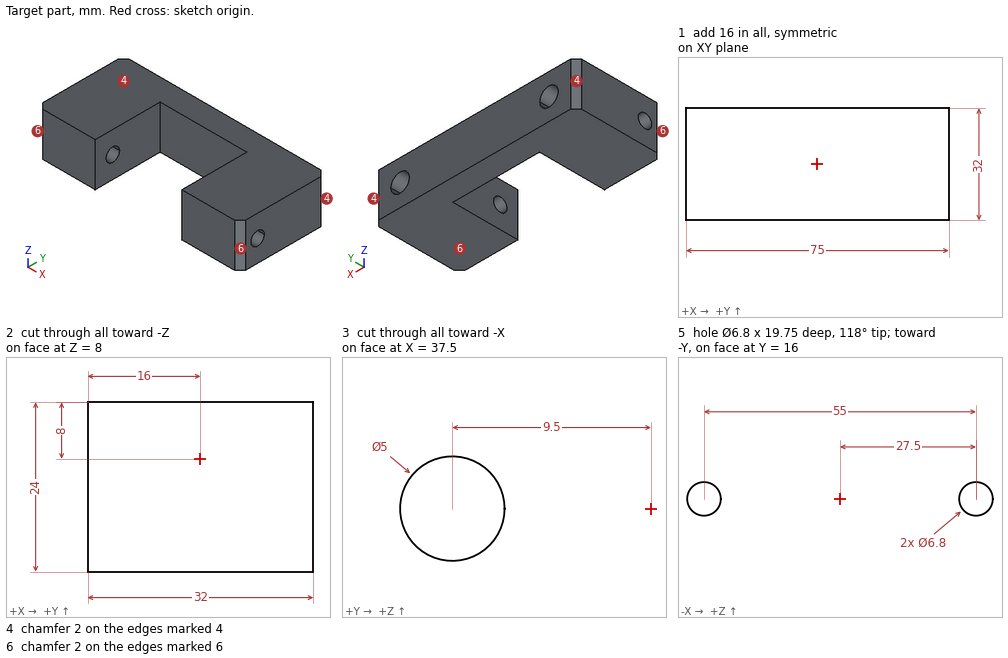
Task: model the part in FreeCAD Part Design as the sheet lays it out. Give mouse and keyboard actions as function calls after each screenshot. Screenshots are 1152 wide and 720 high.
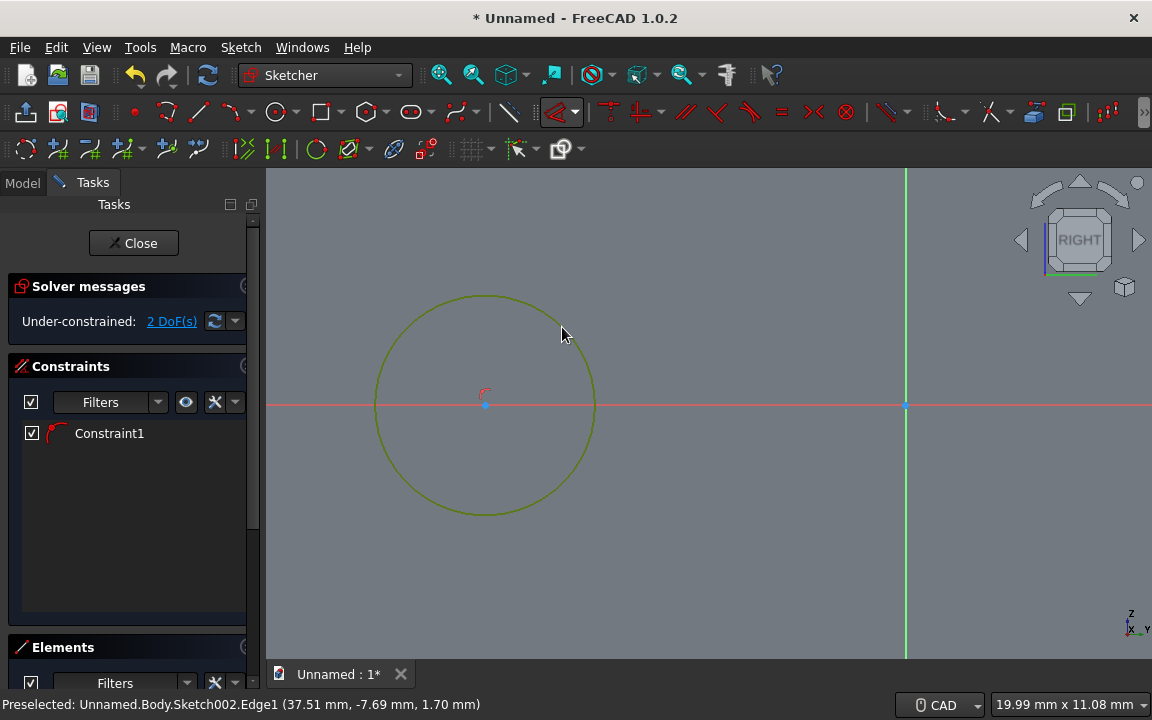
key(k)
key(o)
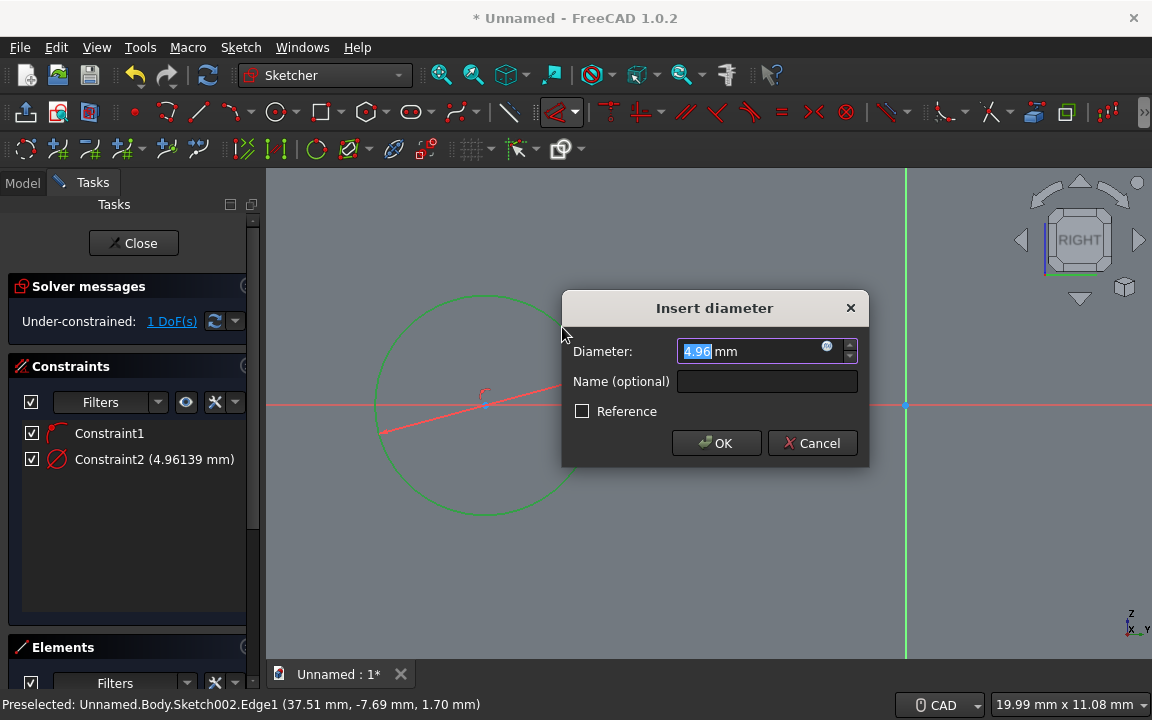
text(5)
key(Return)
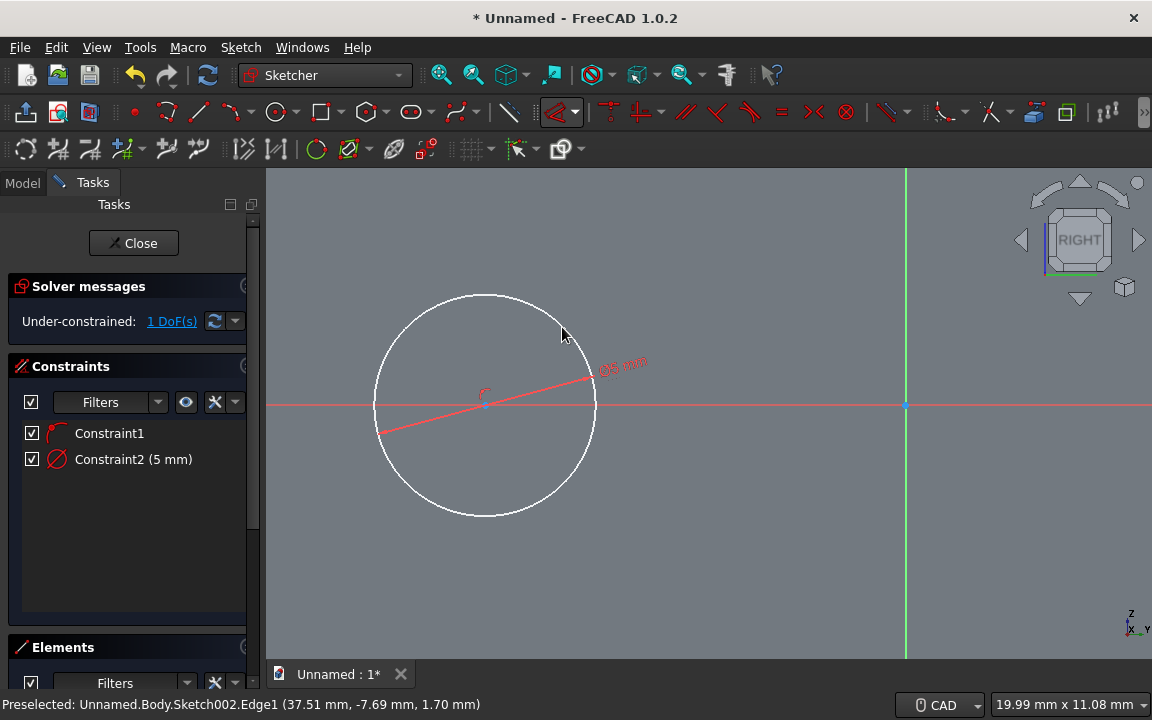
click(485, 405)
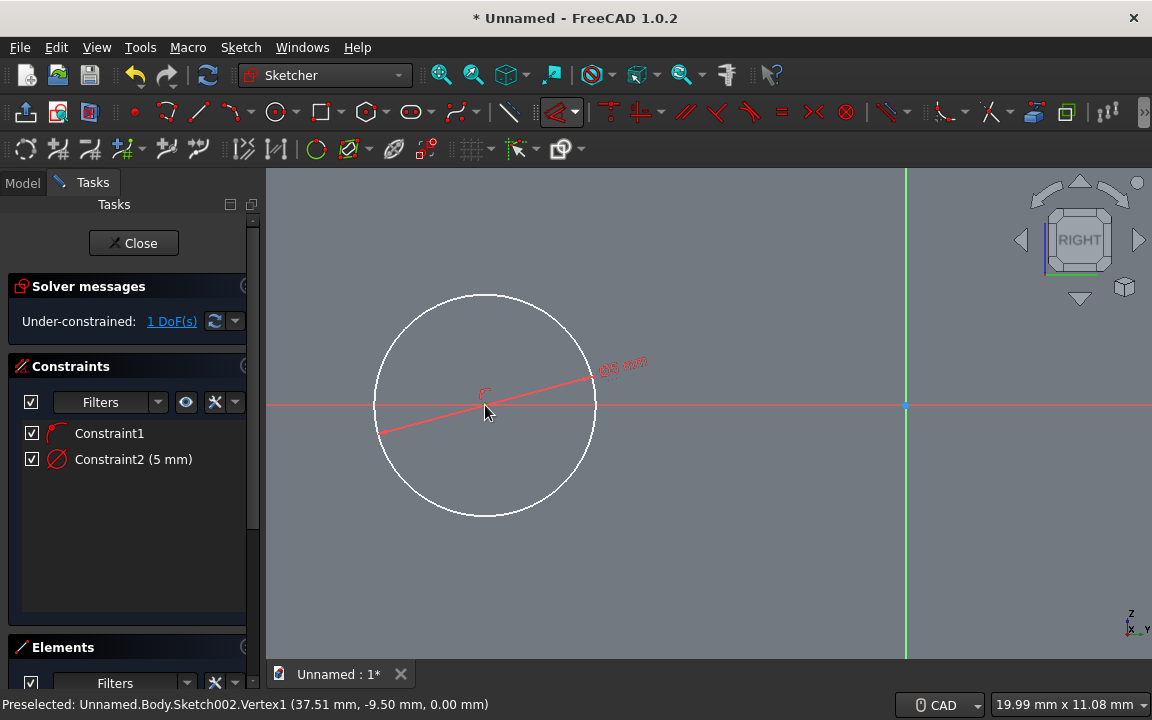
click(578, 112)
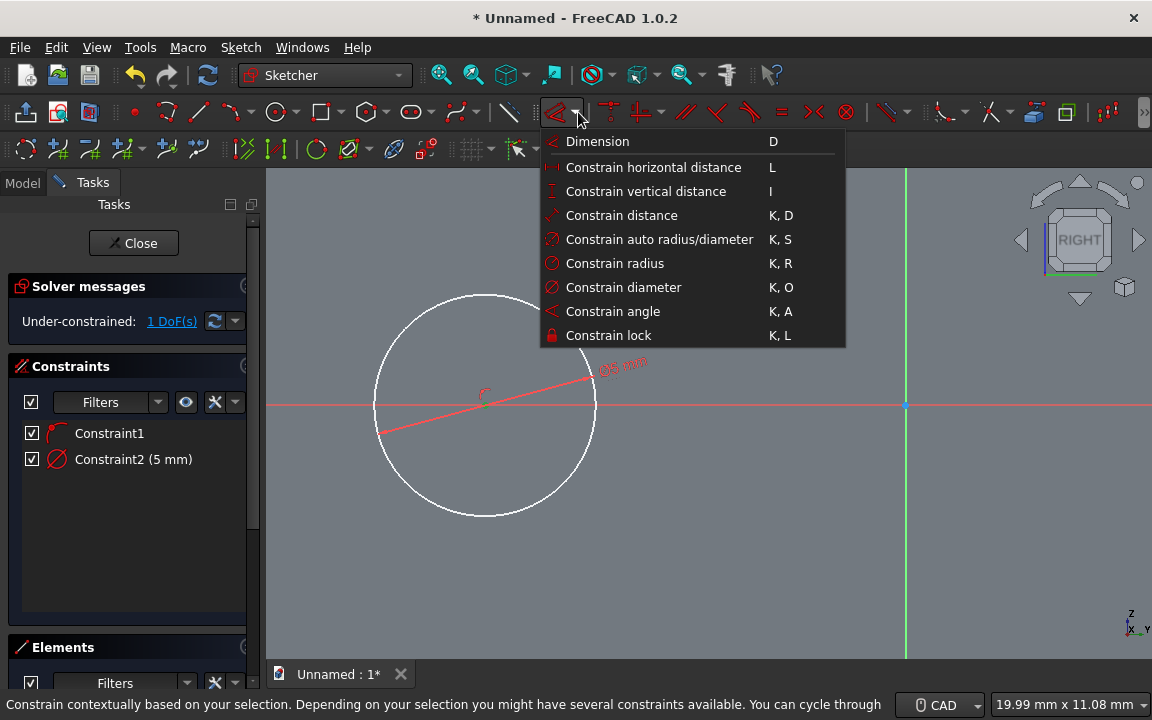
click(693, 167)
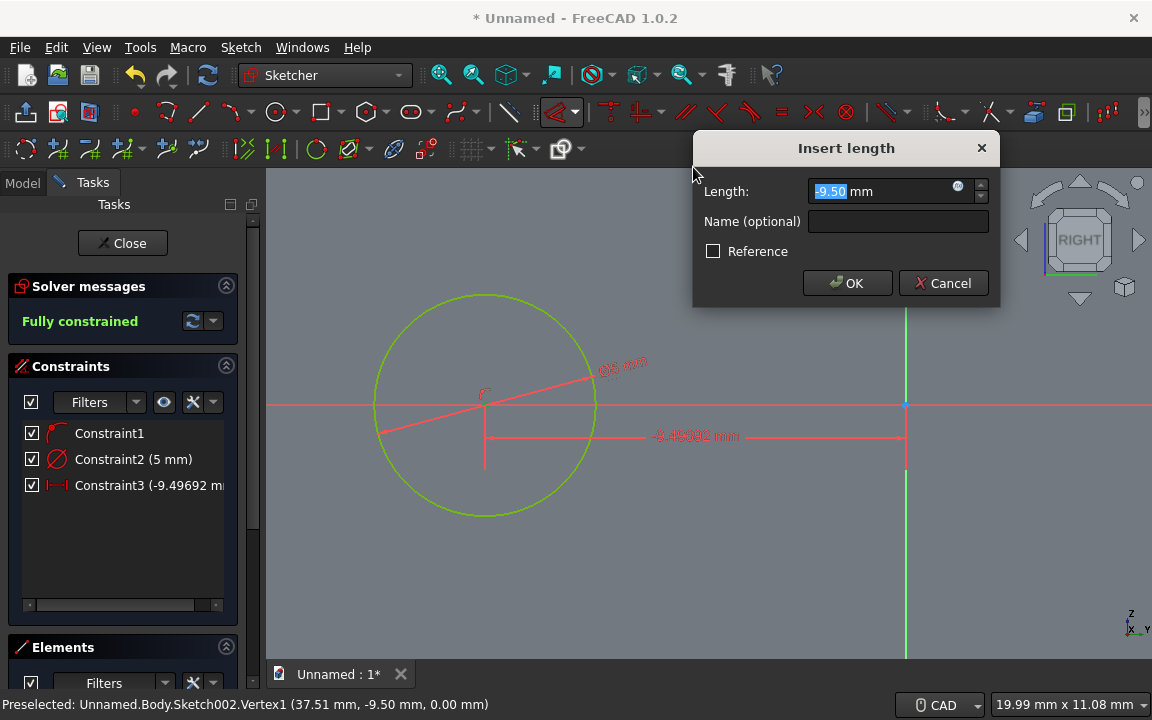
text(-9.5)
key(Return)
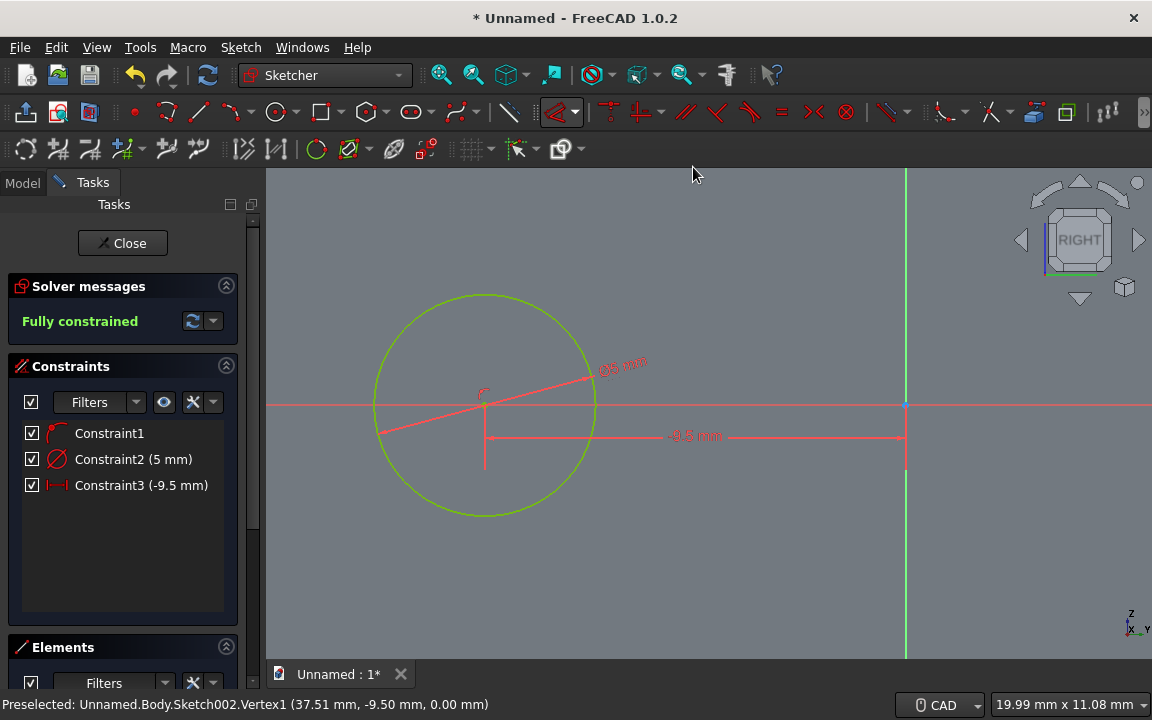
click(123, 243)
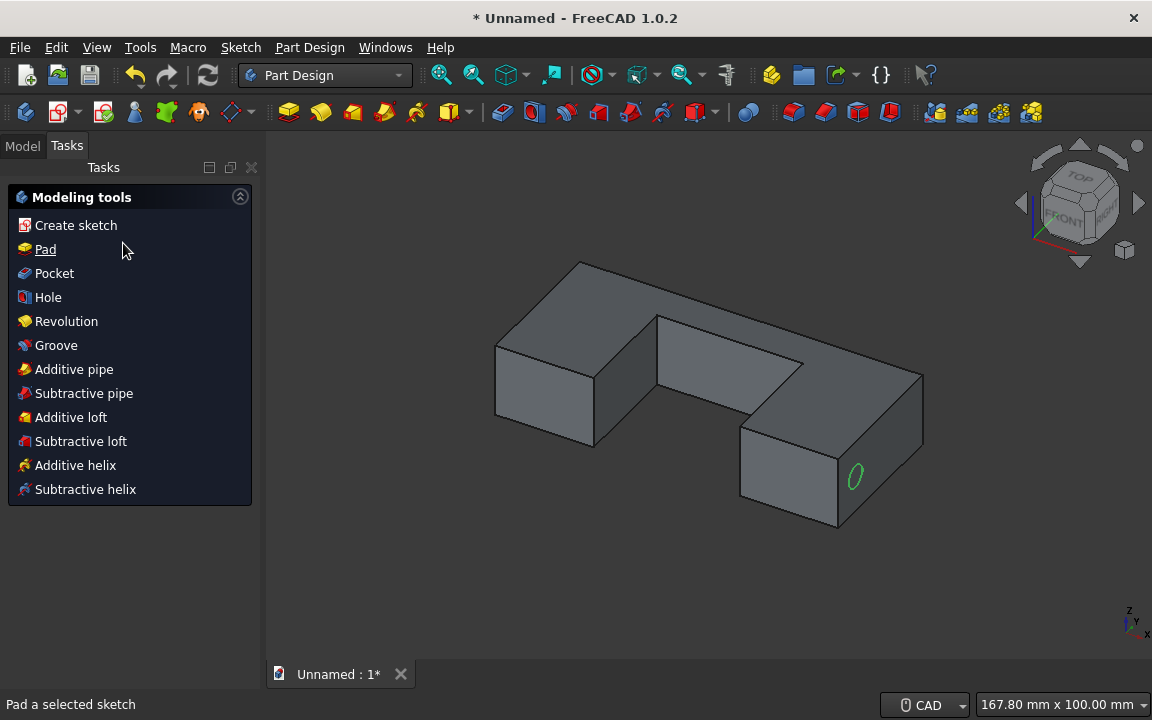
click(504, 112)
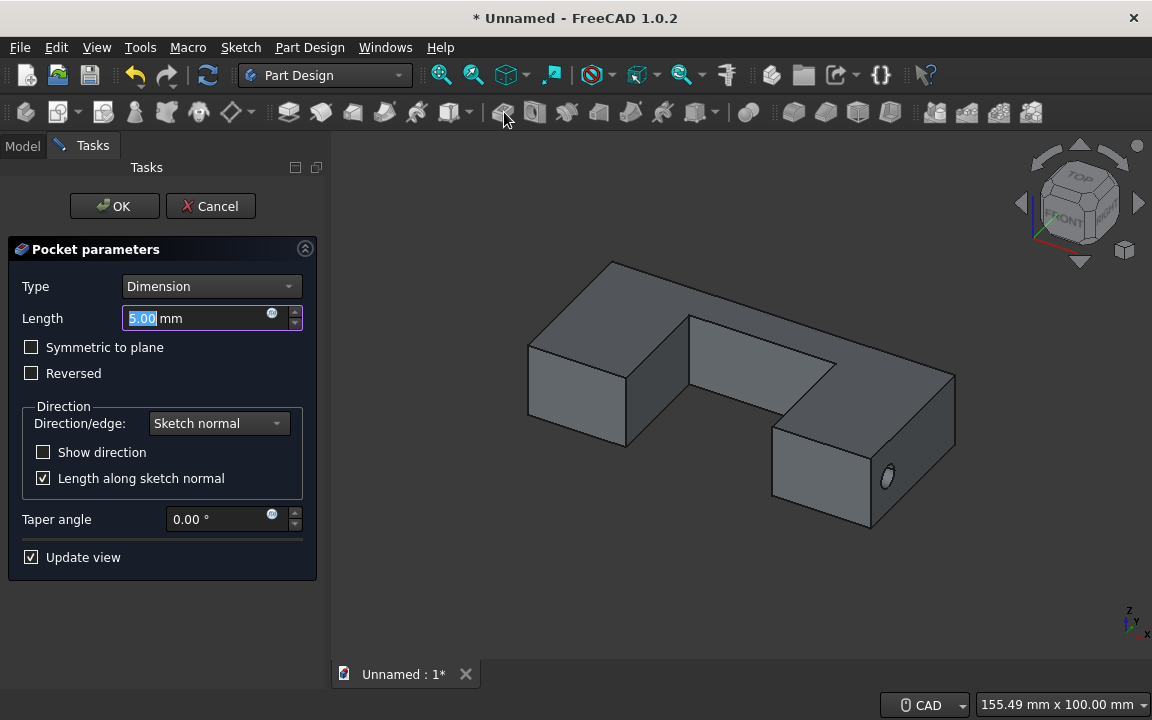
click(212, 286)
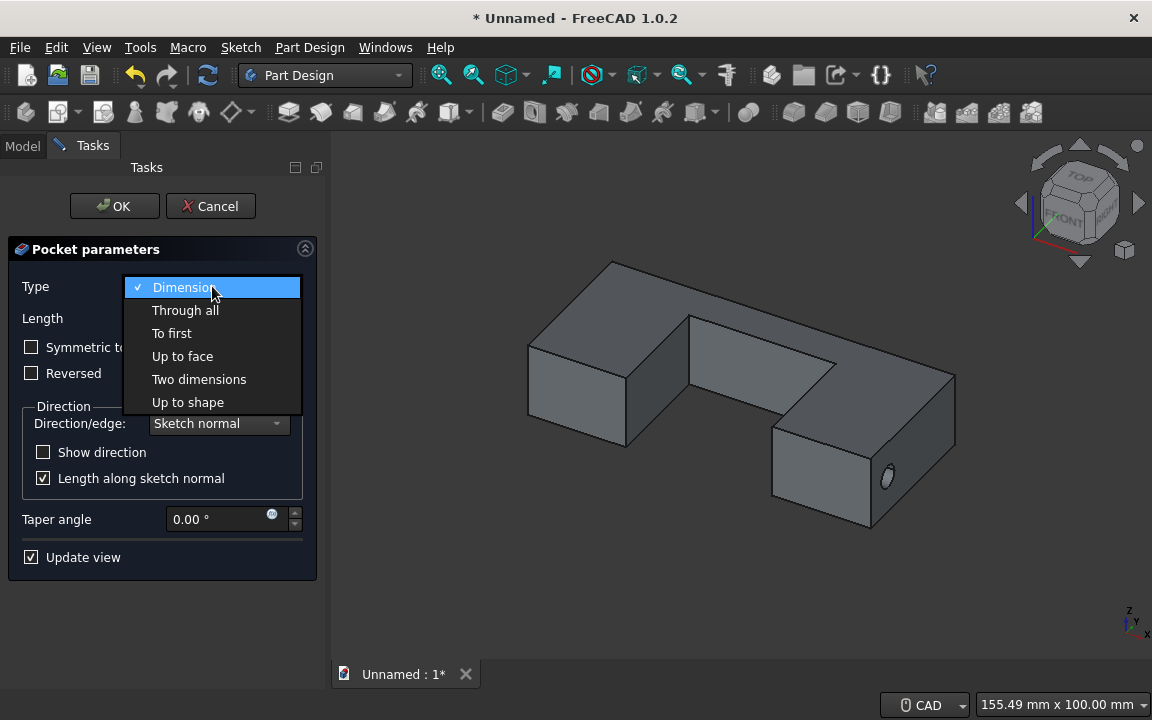
click(212, 310)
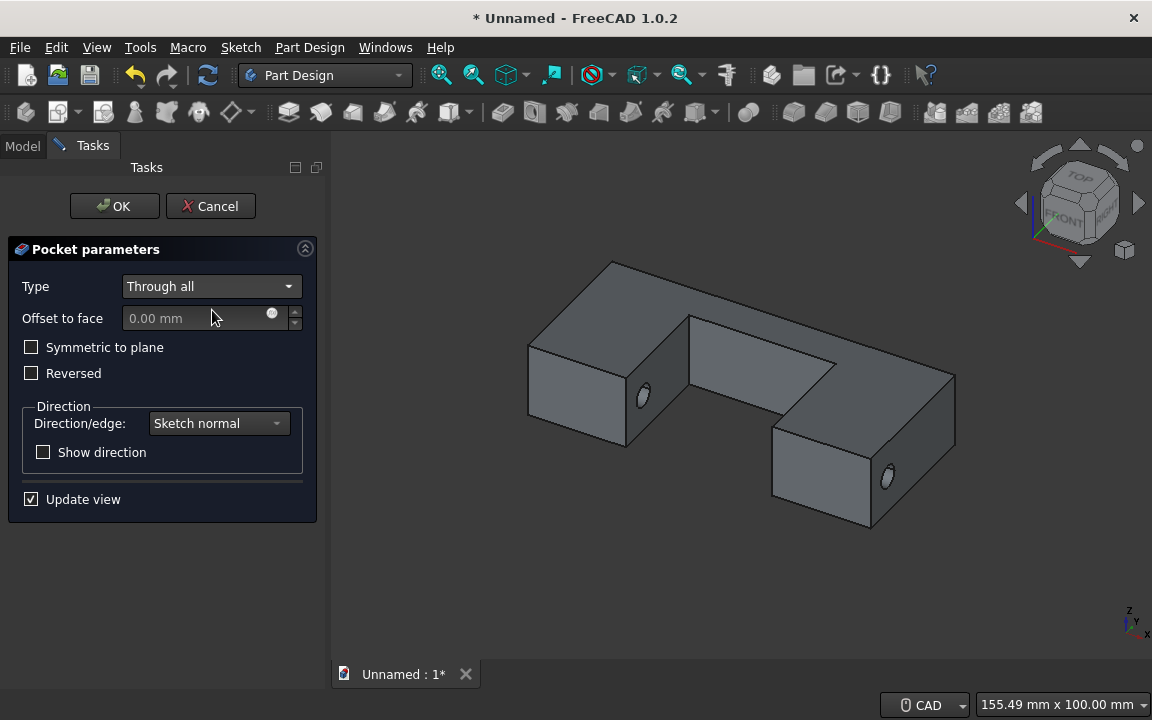
click(115, 206)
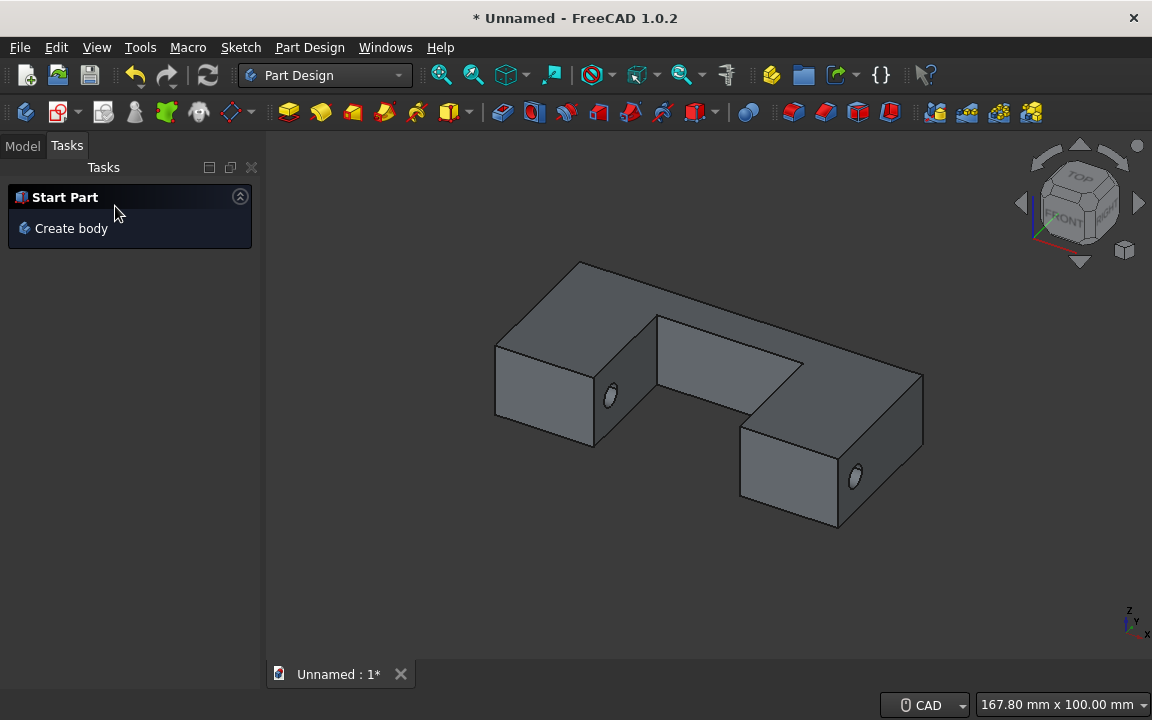
key(0)